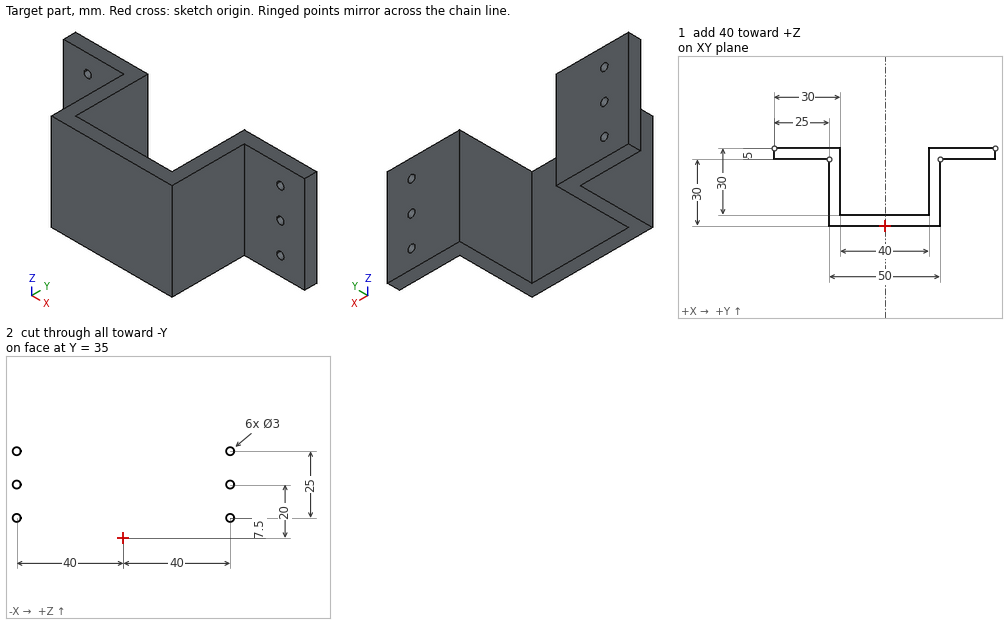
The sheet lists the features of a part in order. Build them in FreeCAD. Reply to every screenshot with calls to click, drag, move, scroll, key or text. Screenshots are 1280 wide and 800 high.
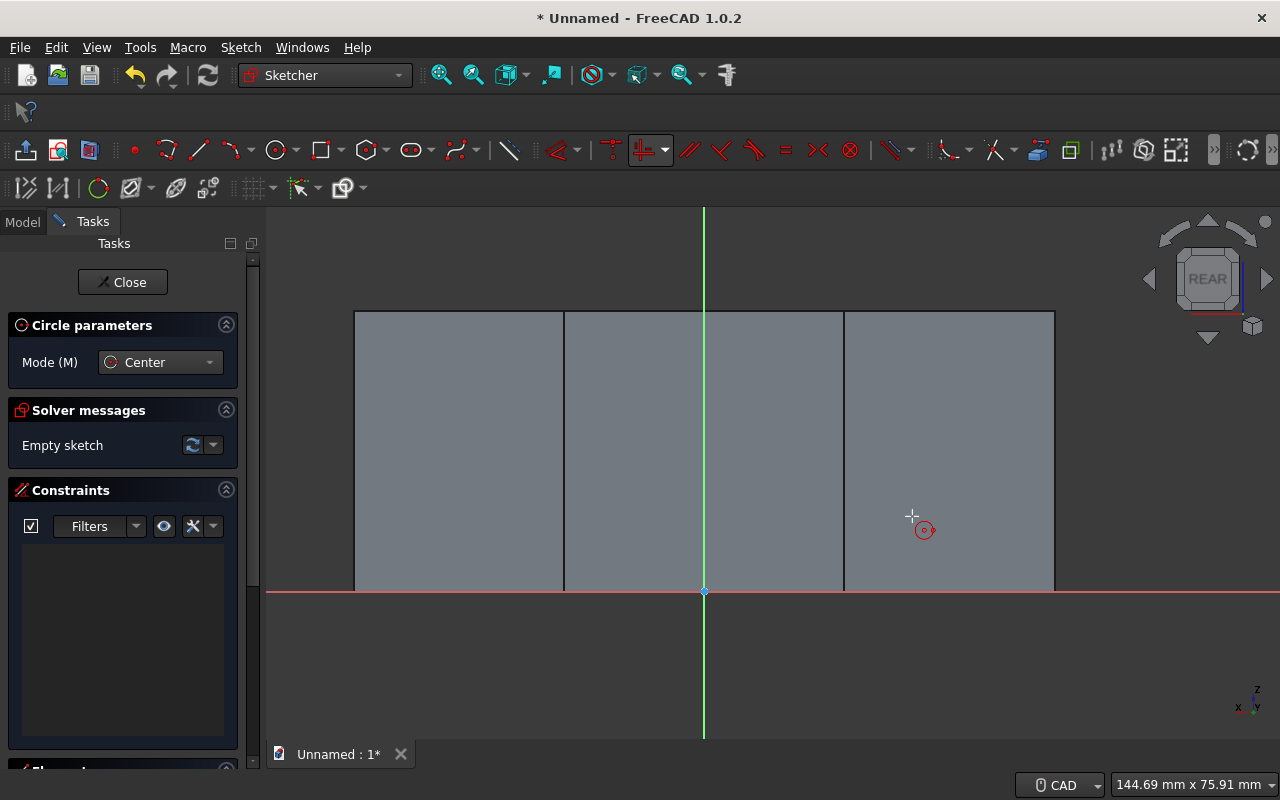
scroll(985, 539, up, 4)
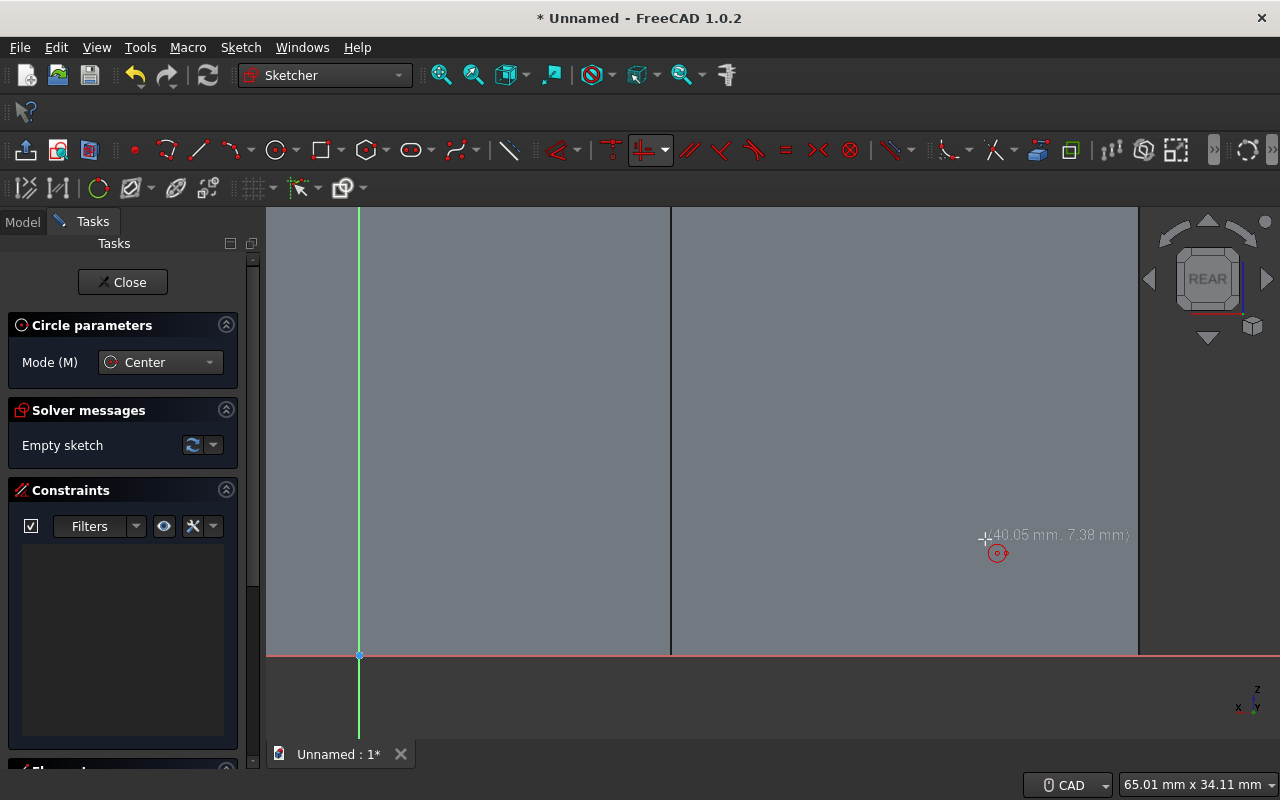
click(983, 539)
move(1000, 522)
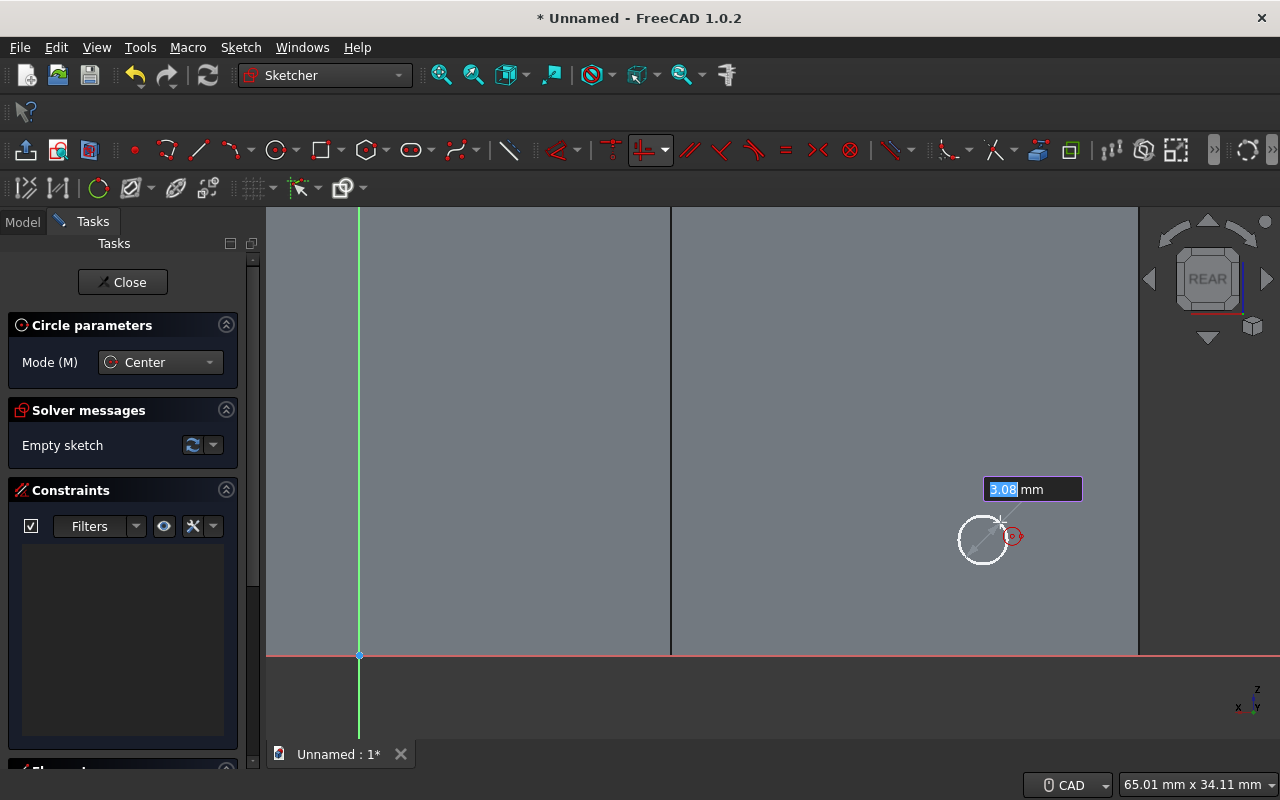
text(3)
key(Return)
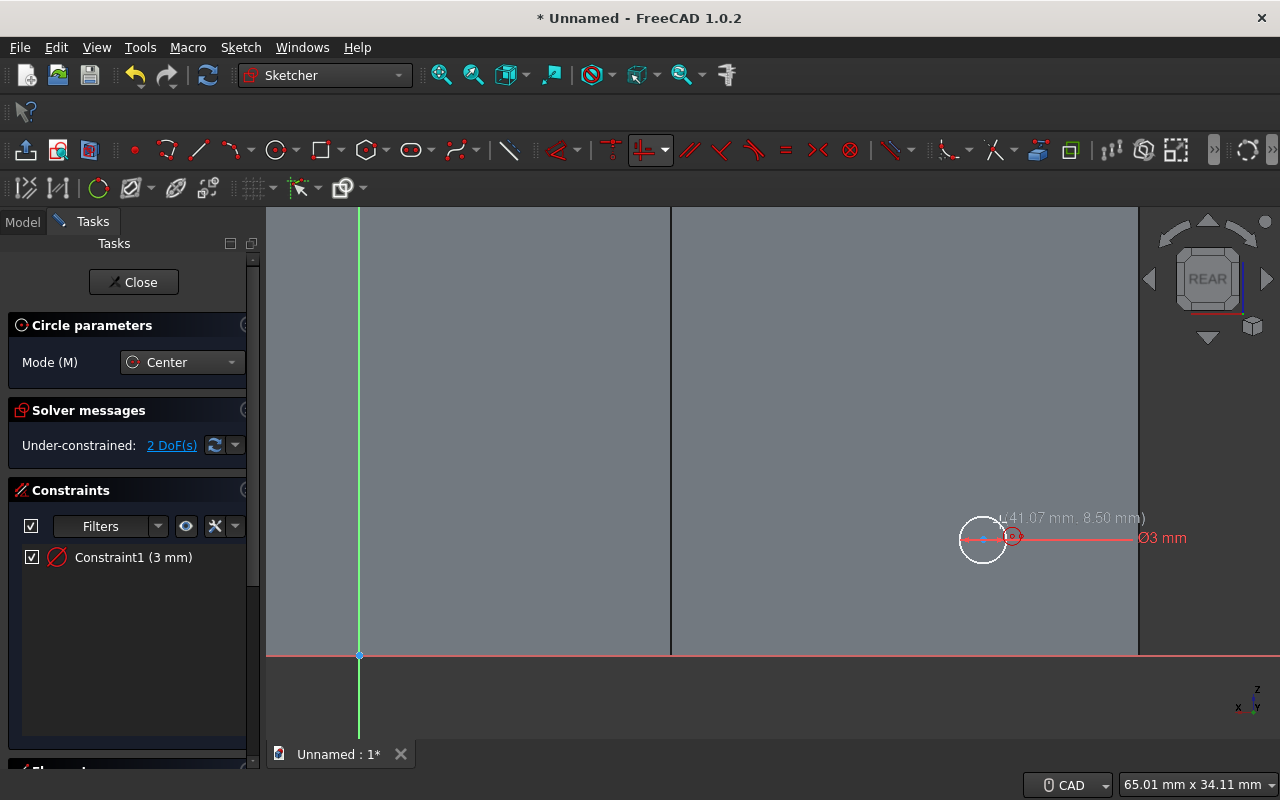
click(983, 344)
move(1000, 327)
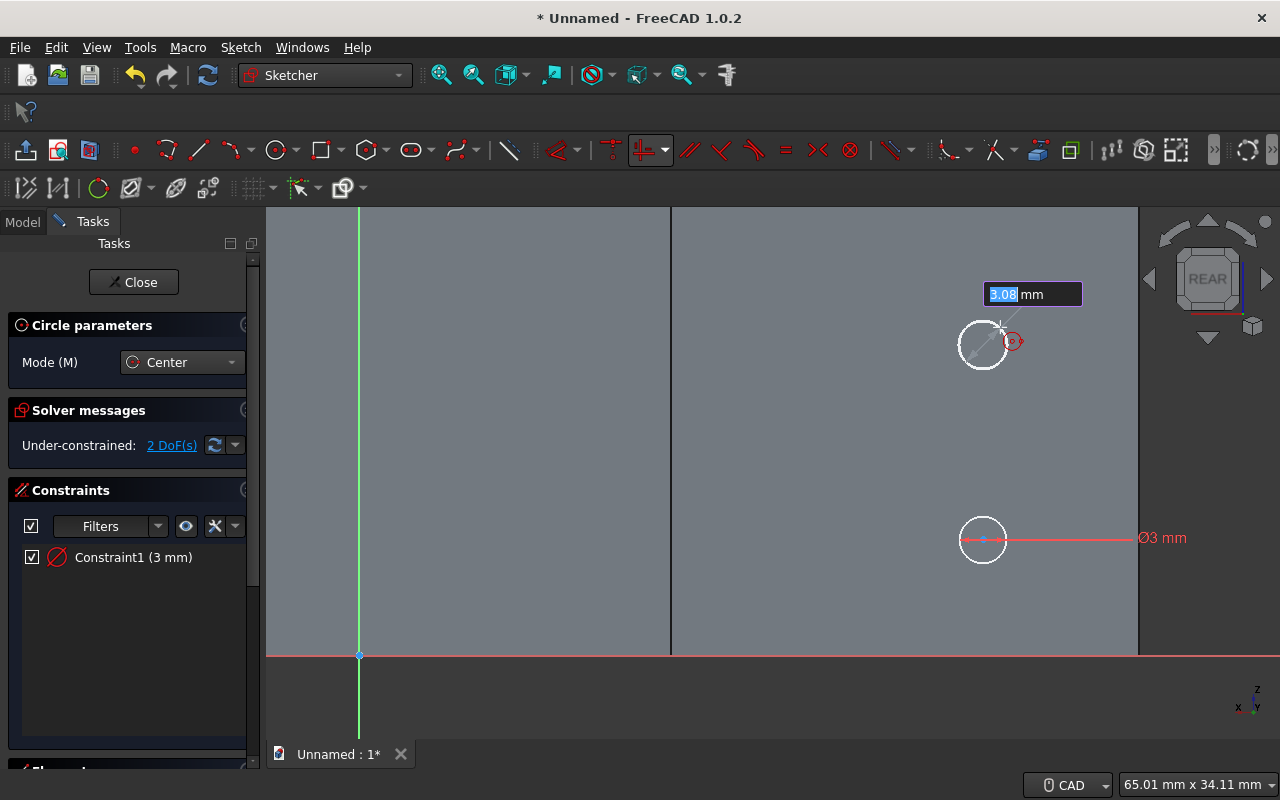
text(3)
key(Return)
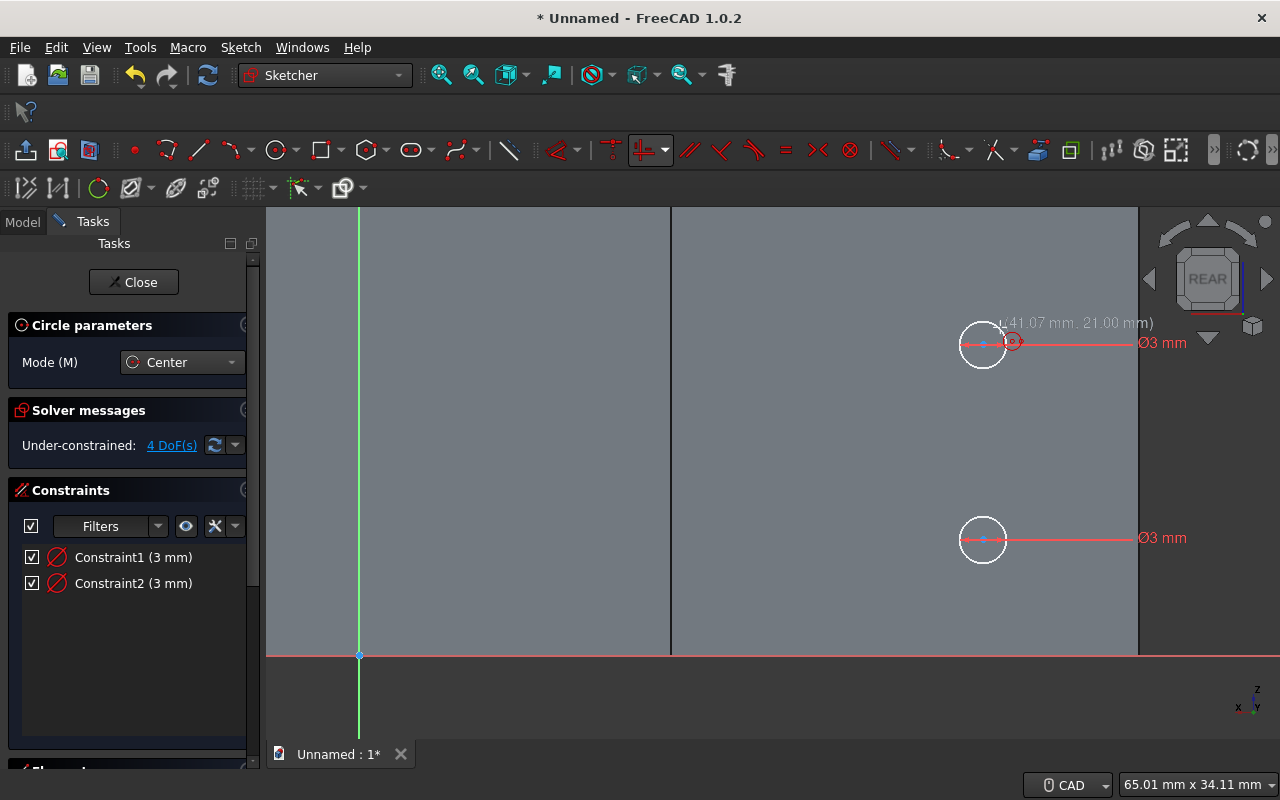
scroll(986, 540, down, 4)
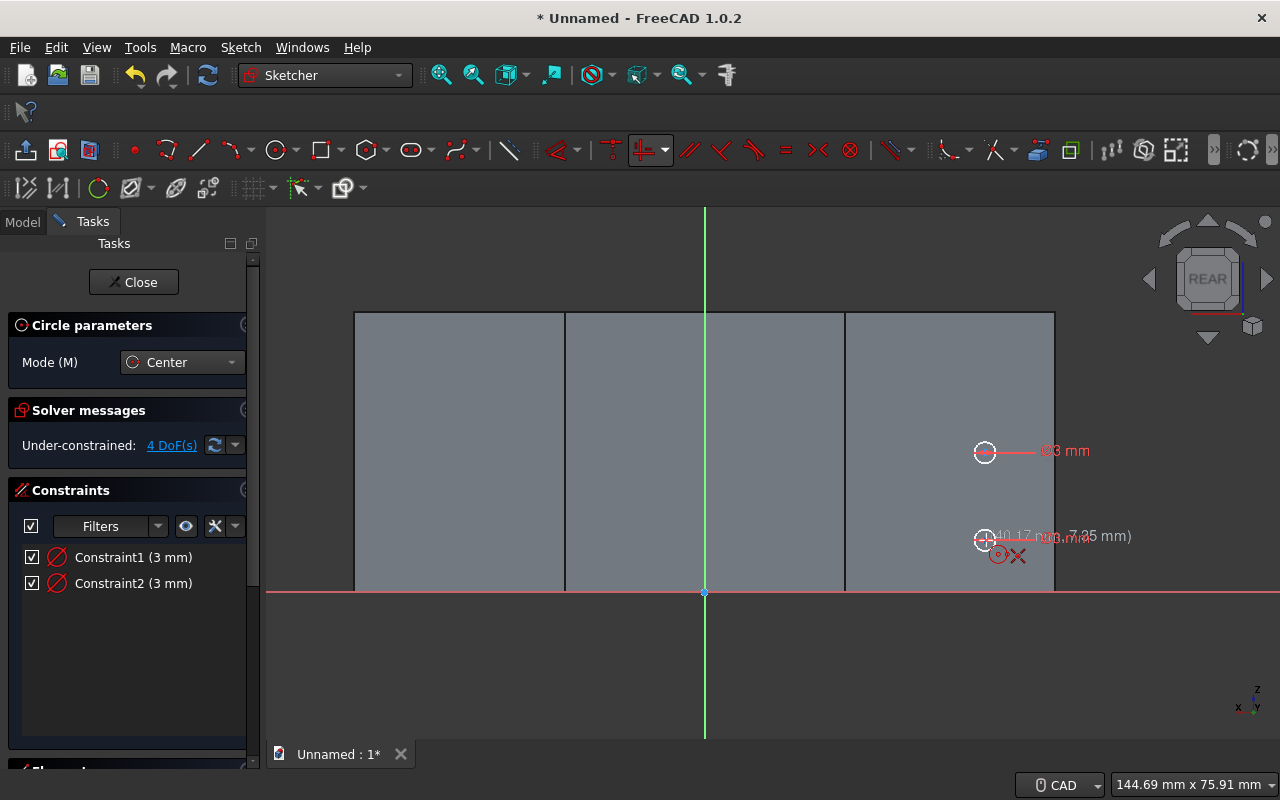
scroll(985, 365, up, 4)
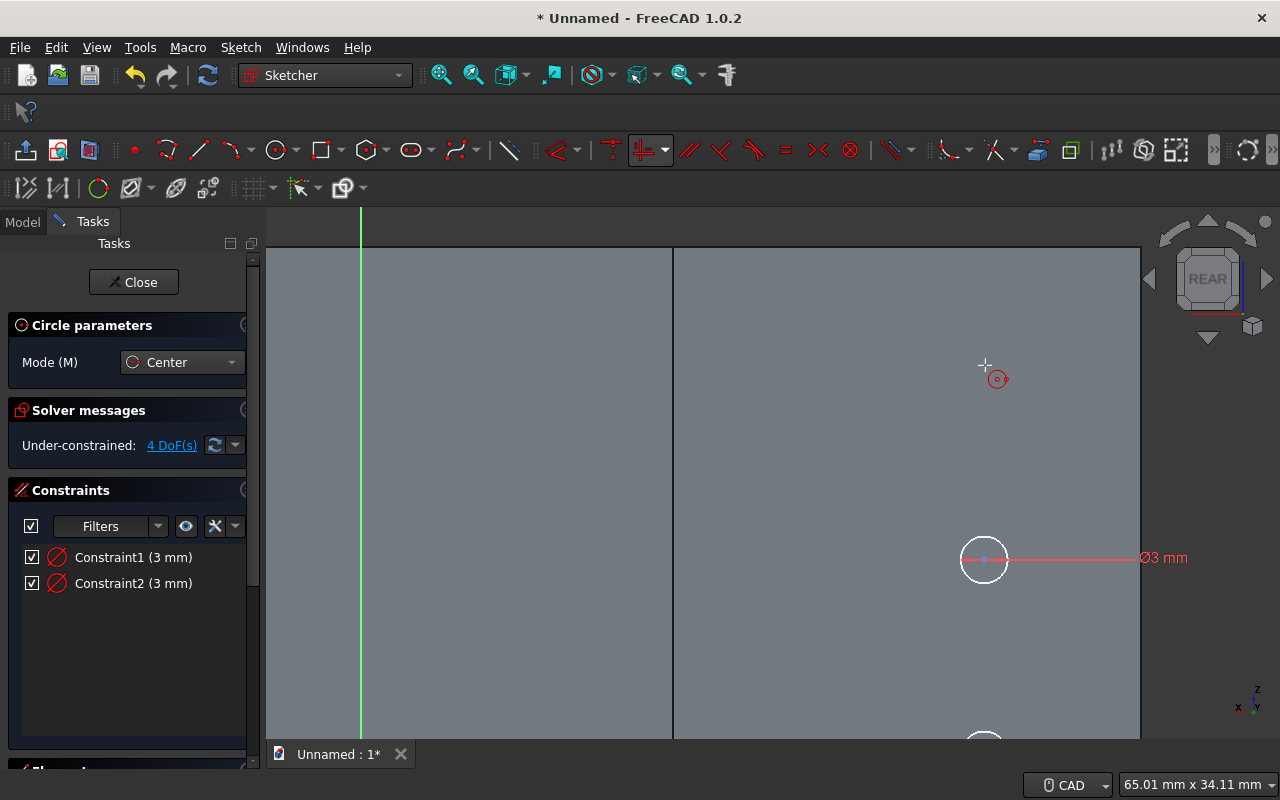
click(985, 364)
move(1001, 347)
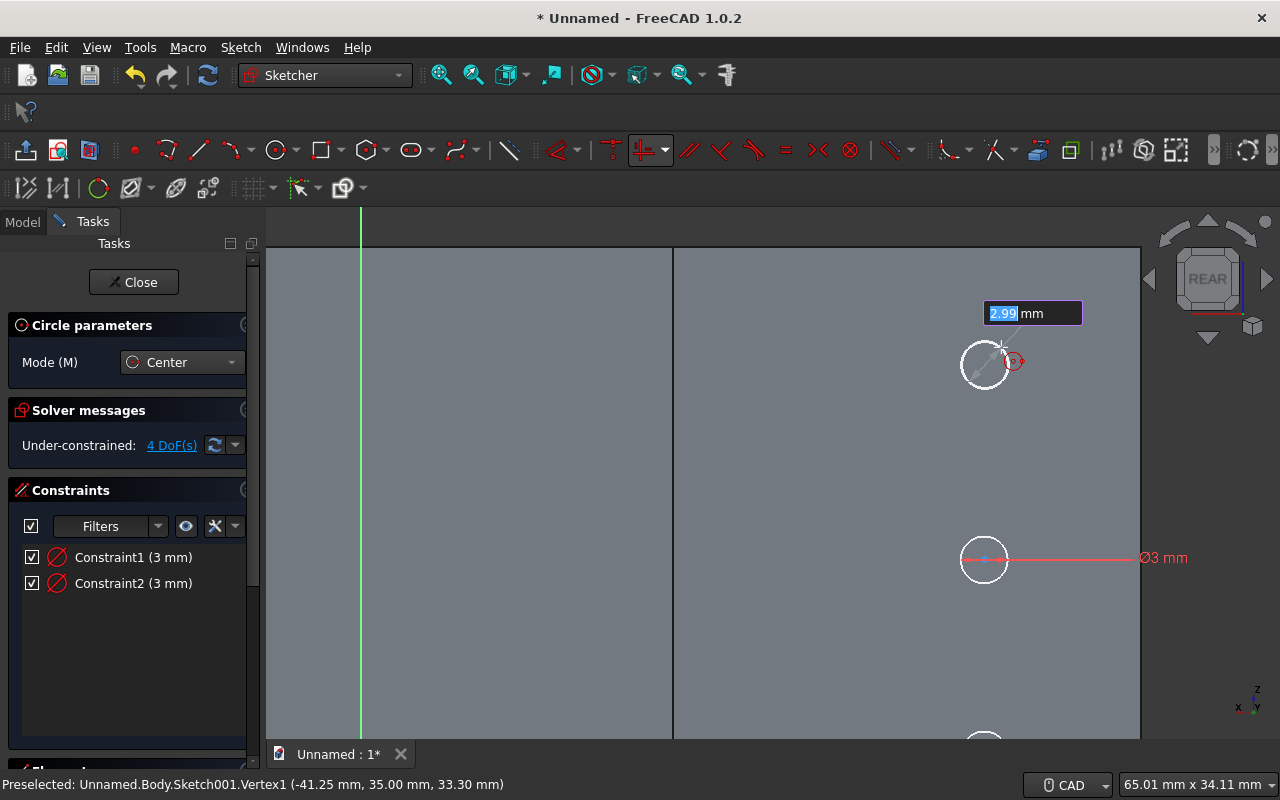
text(3)
key(Return)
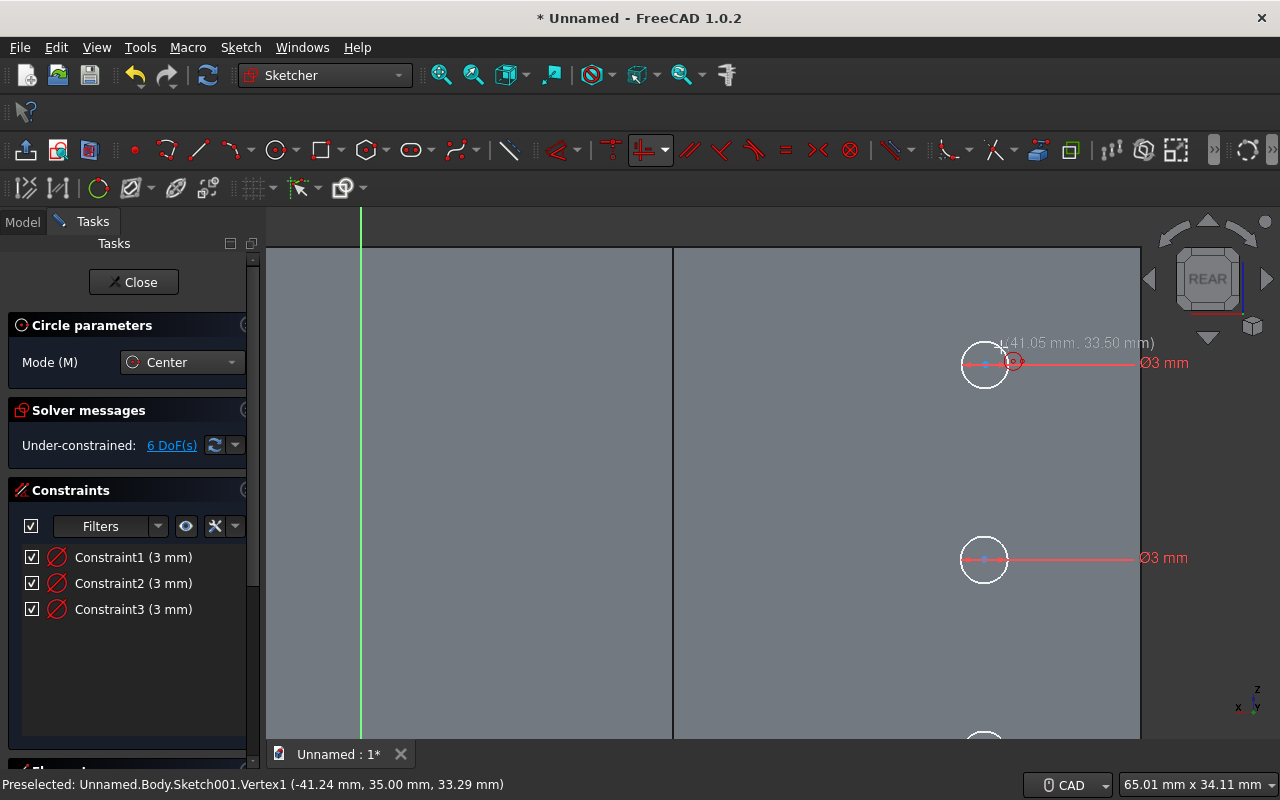
scroll(985, 365, down, 4)